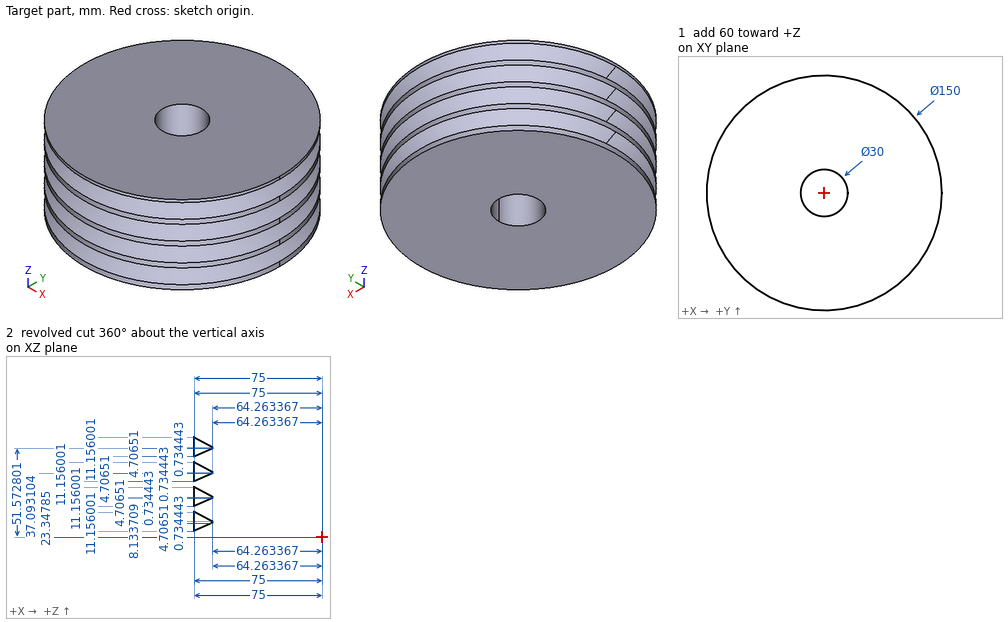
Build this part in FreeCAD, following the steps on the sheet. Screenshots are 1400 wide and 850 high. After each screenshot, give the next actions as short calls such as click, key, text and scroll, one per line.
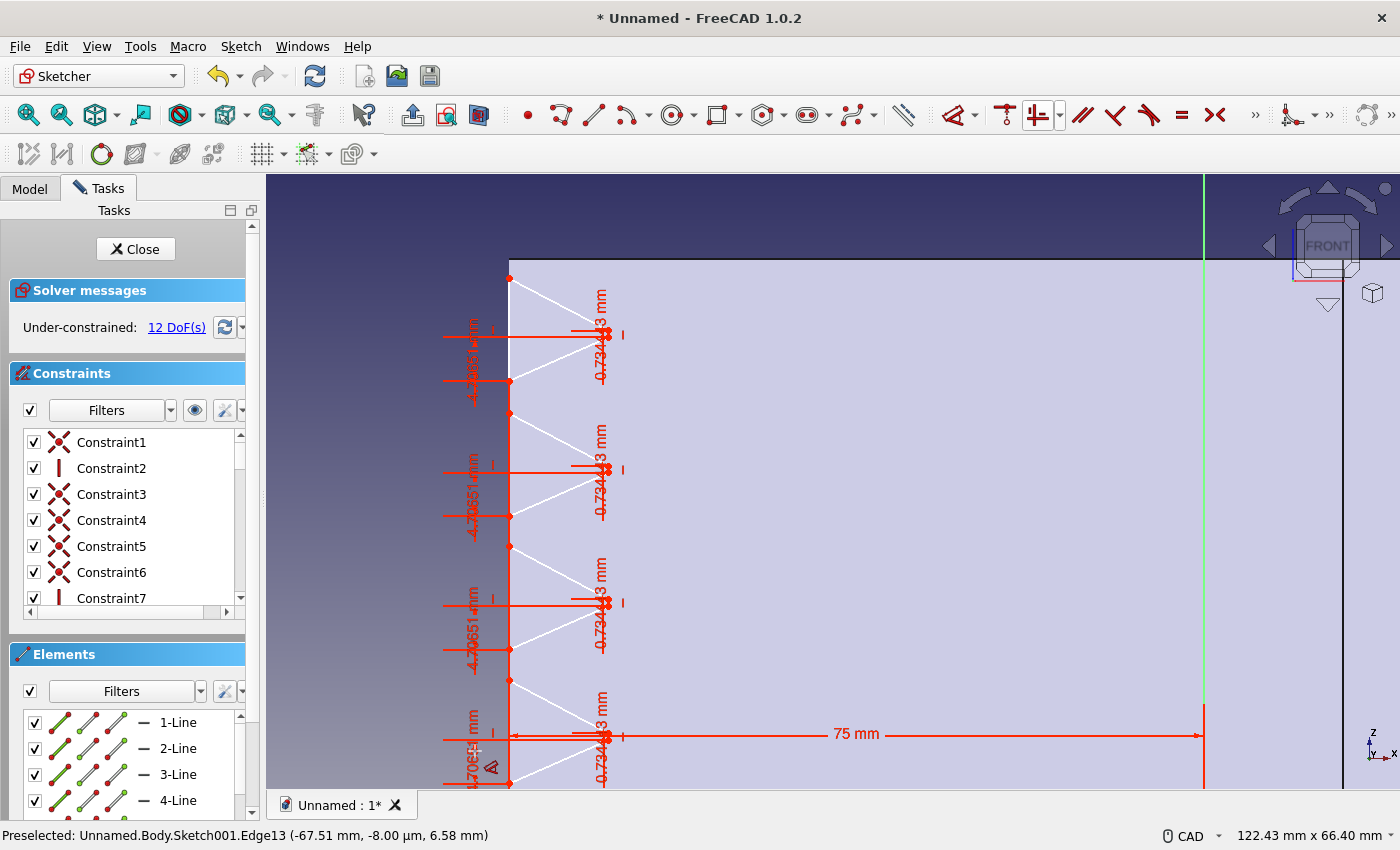
click(509, 350)
click(475, 330)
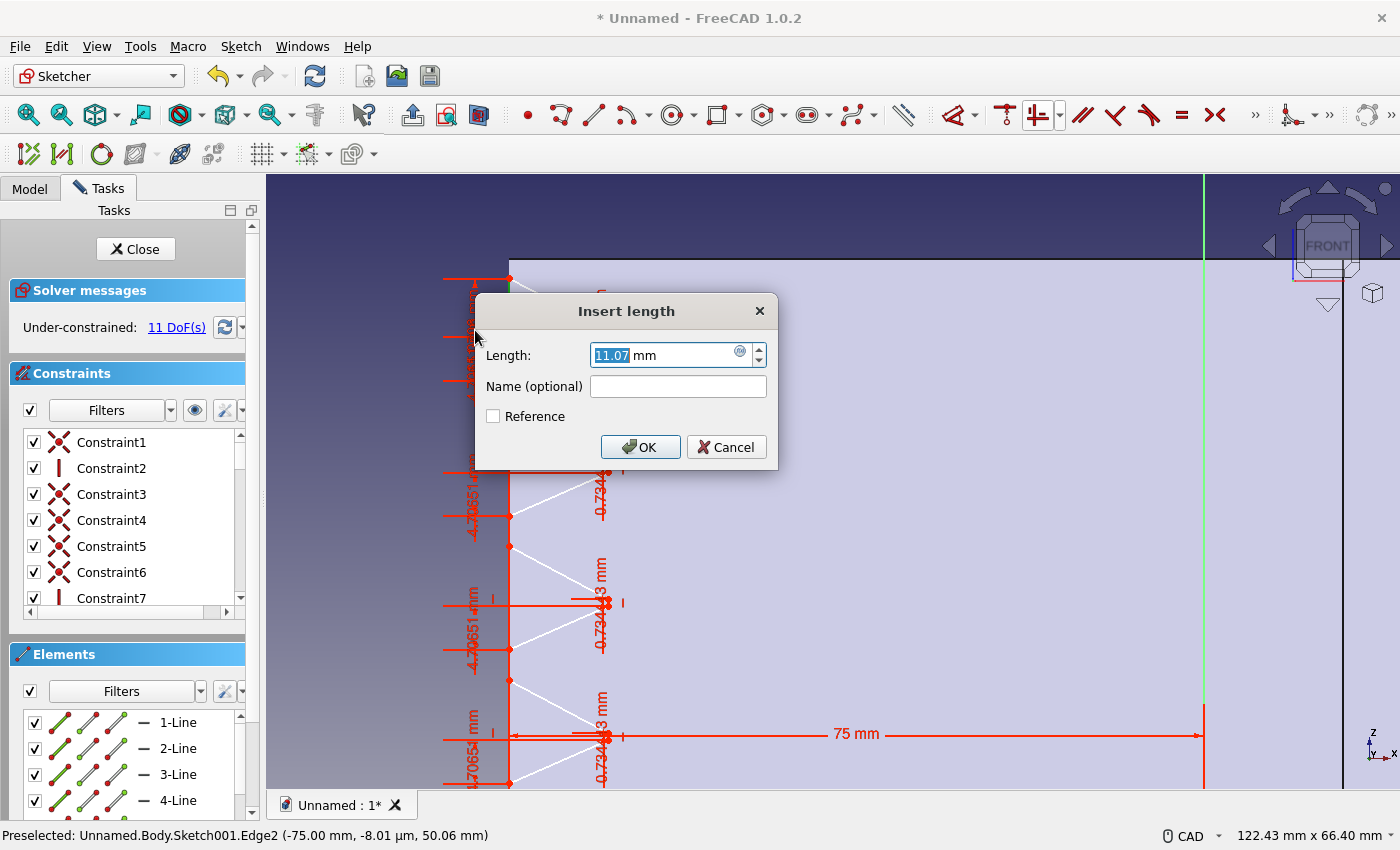
text(11.156001)
key(Return)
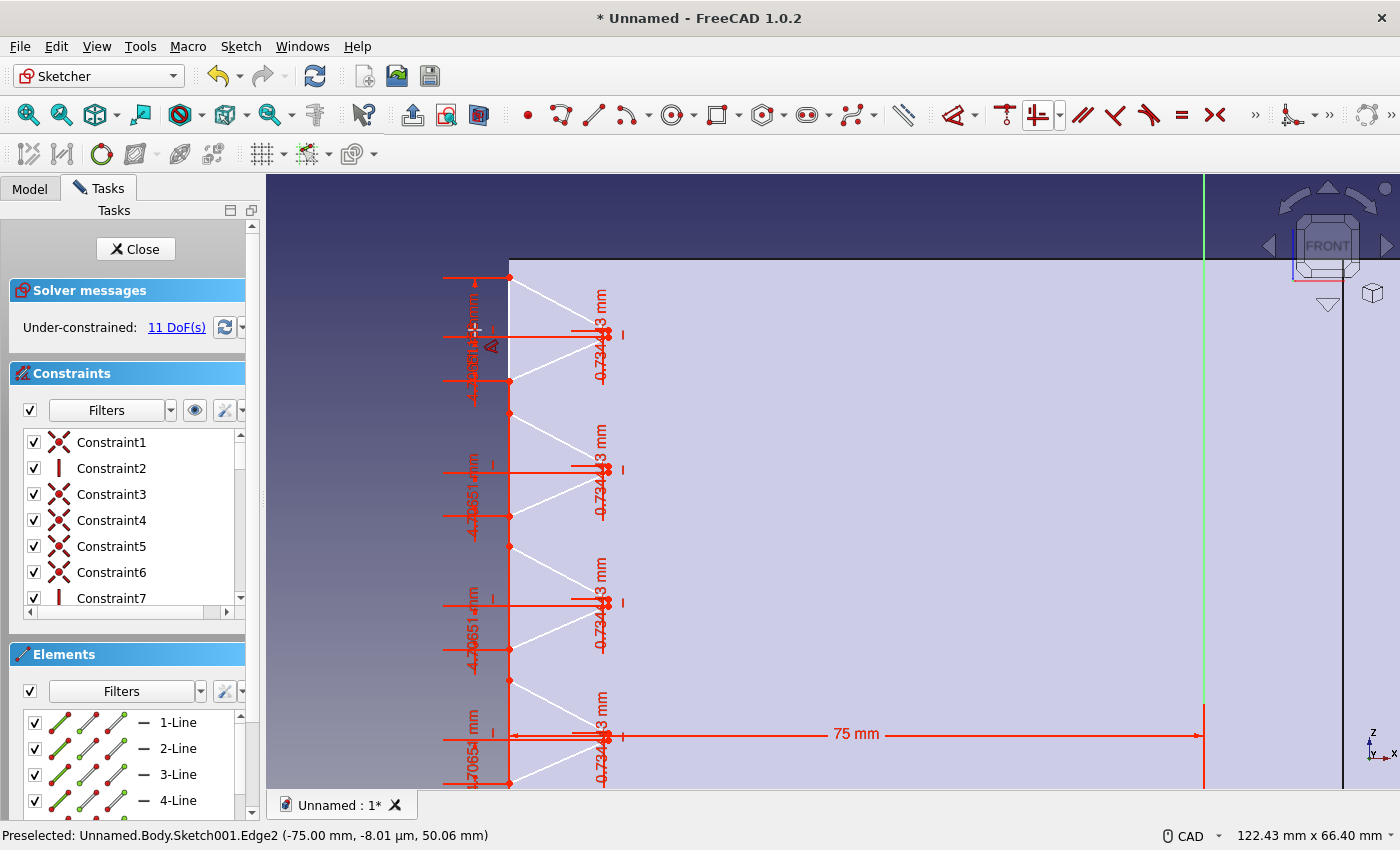
click(509, 486)
click(475, 465)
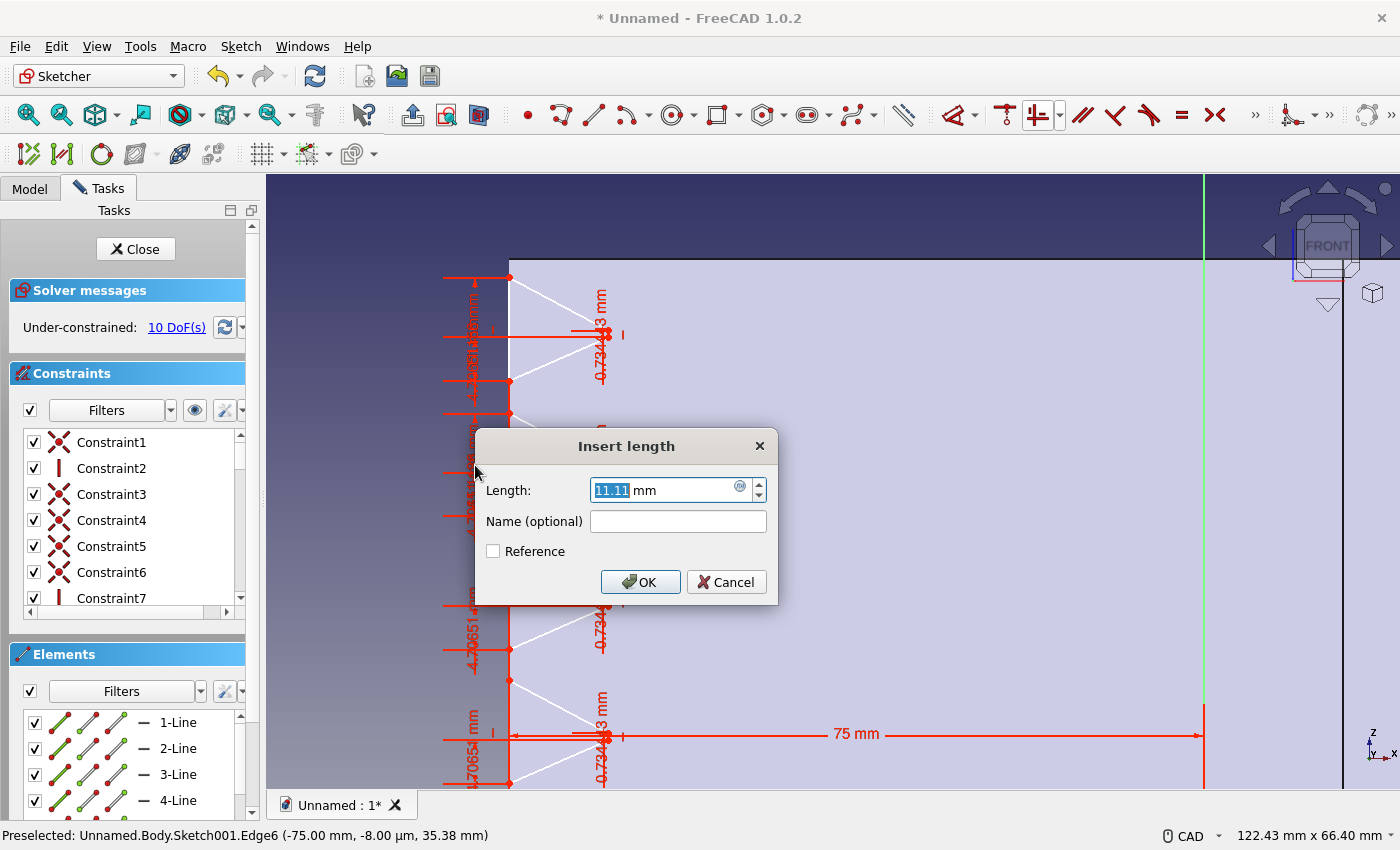
text(11.156001)
key(Return)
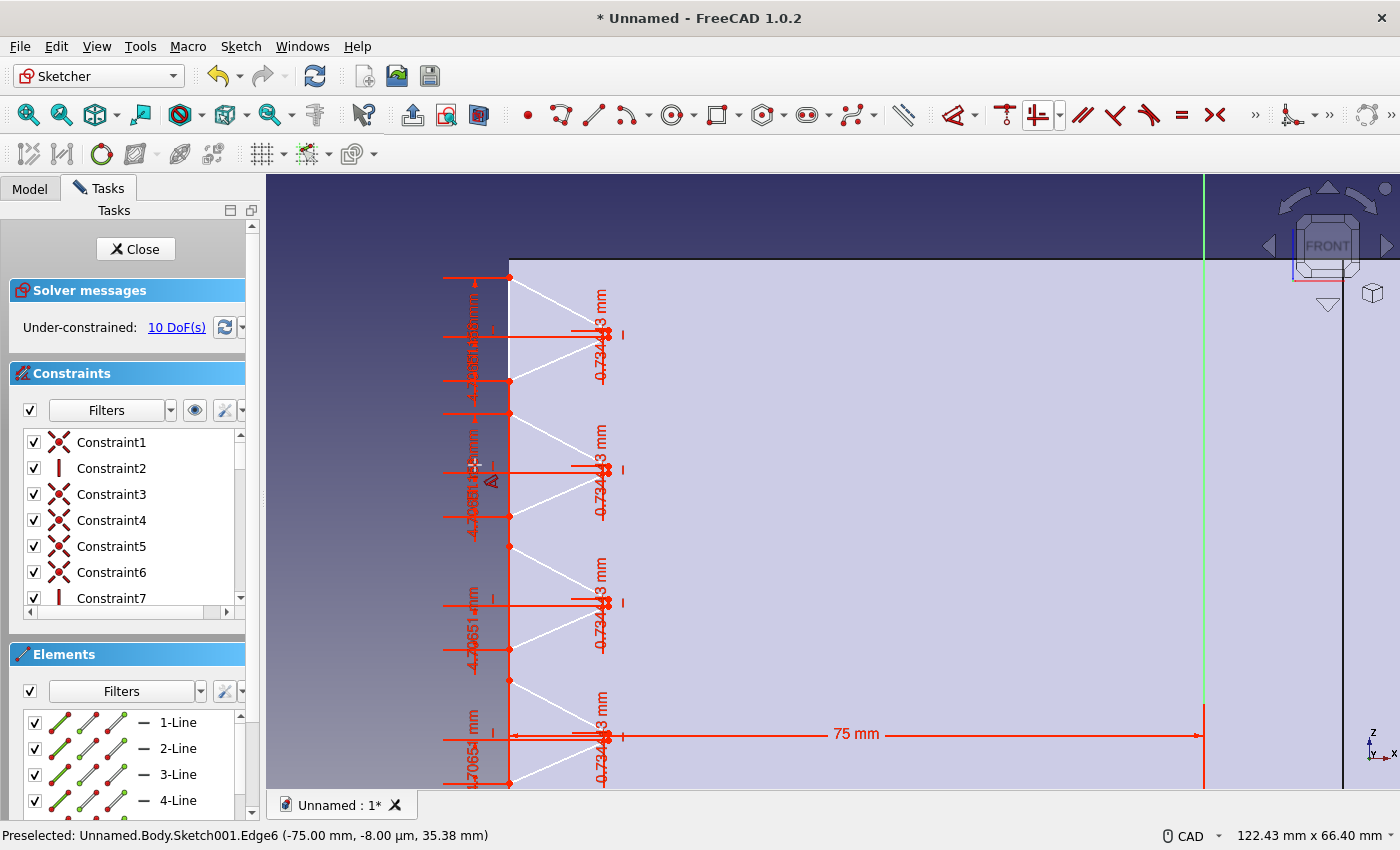
click(509, 619)
click(475, 598)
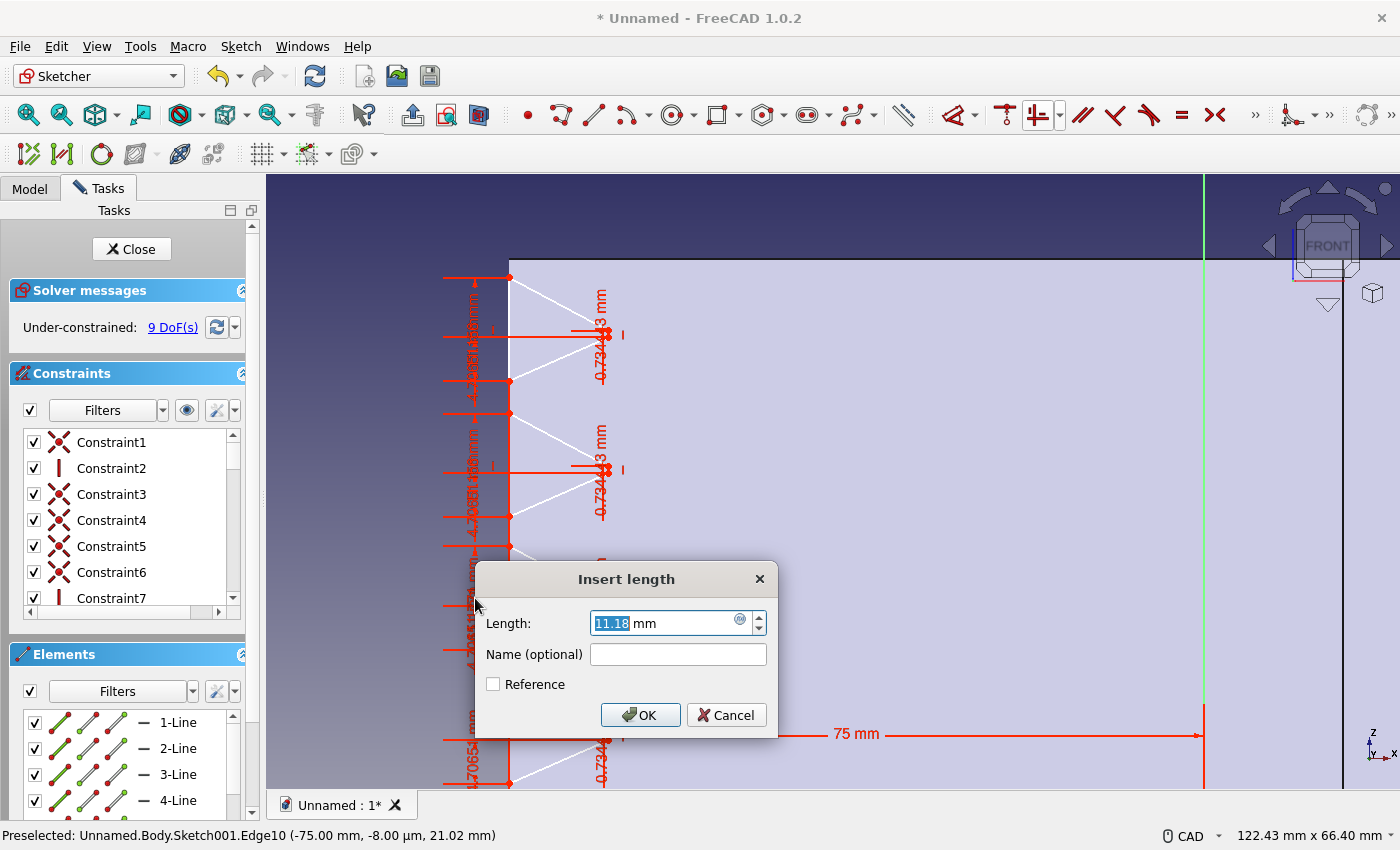
text(11.156001)
key(Return)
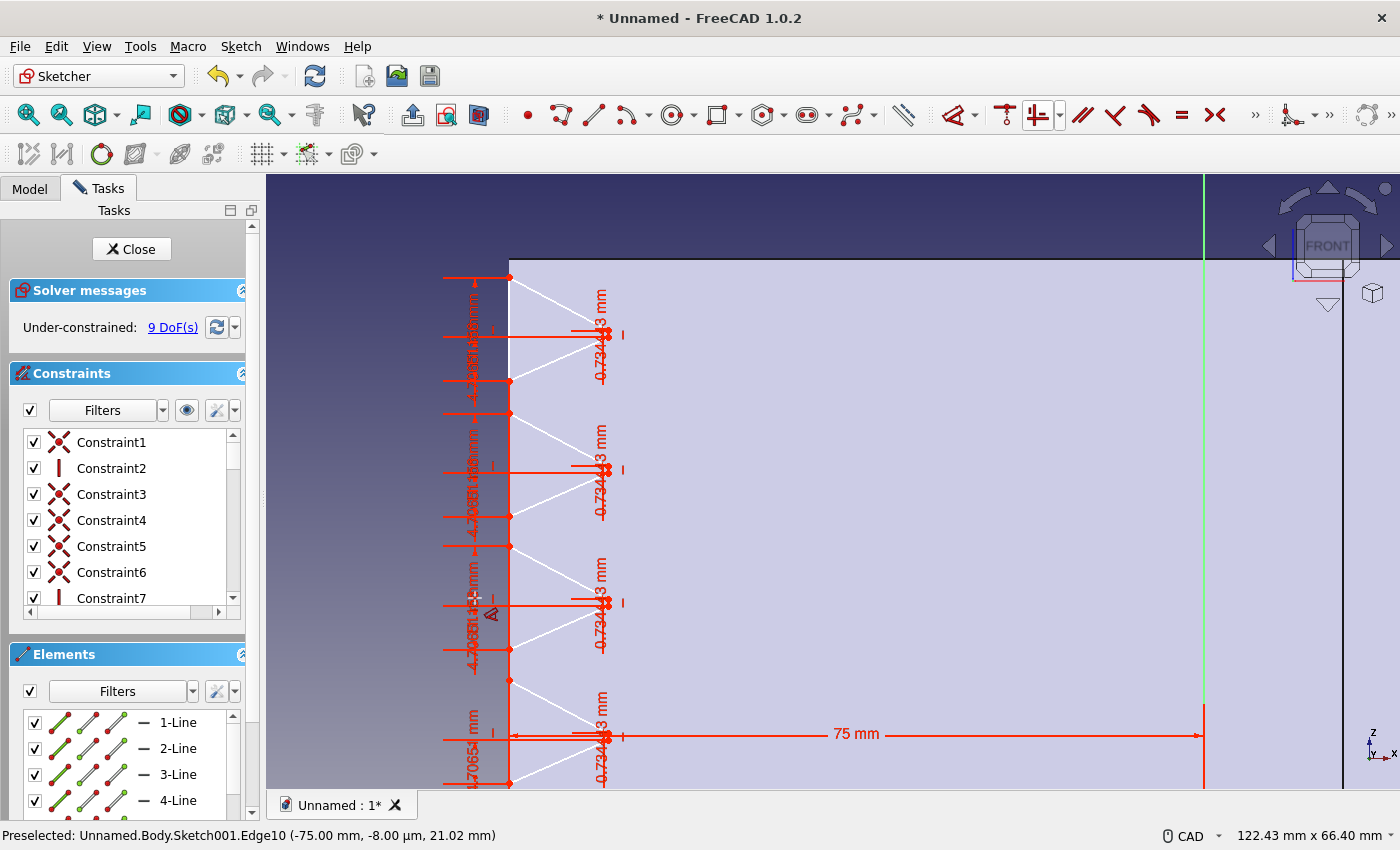
click(509, 753)
click(475, 721)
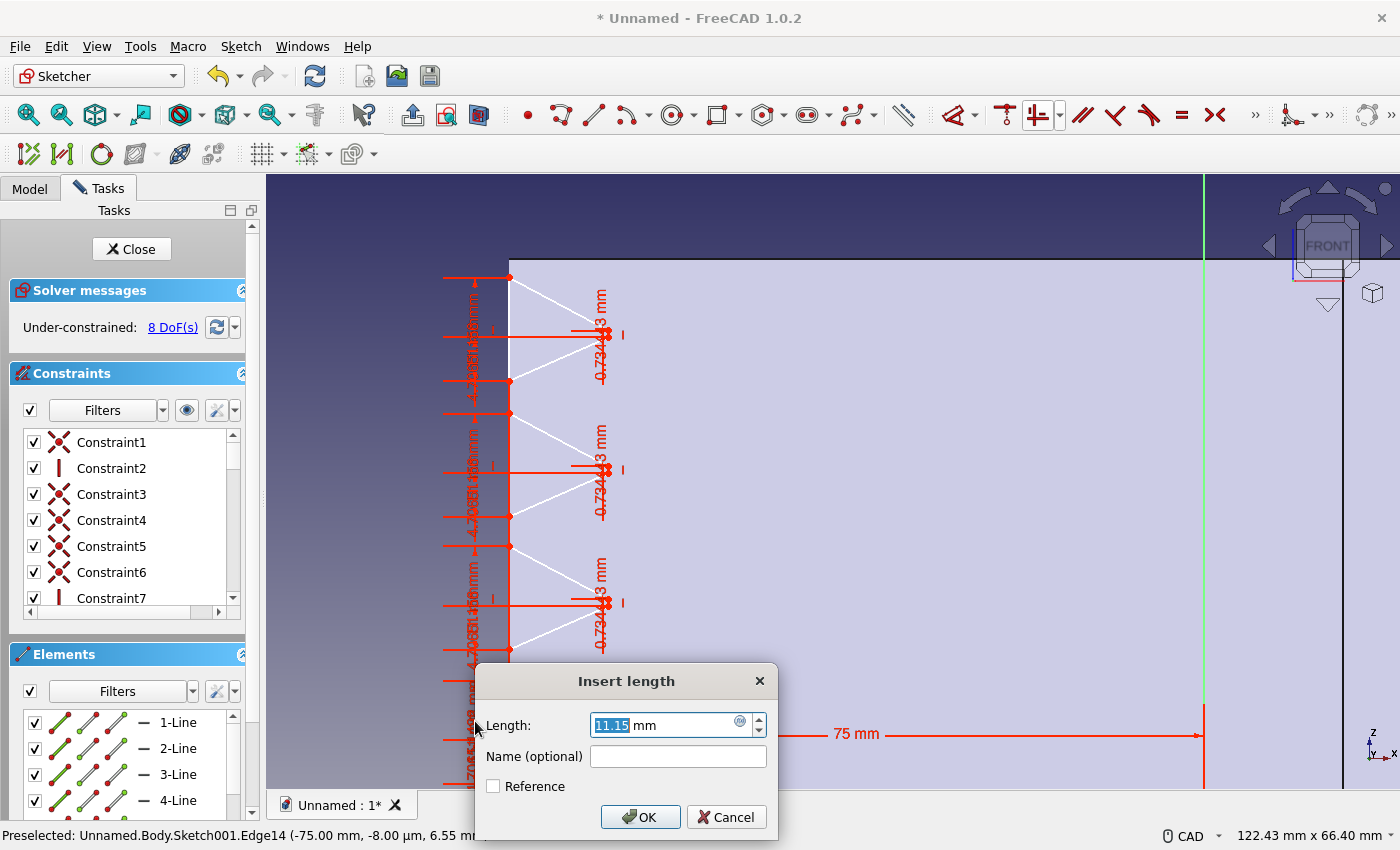
text(11.156001)
key(Return)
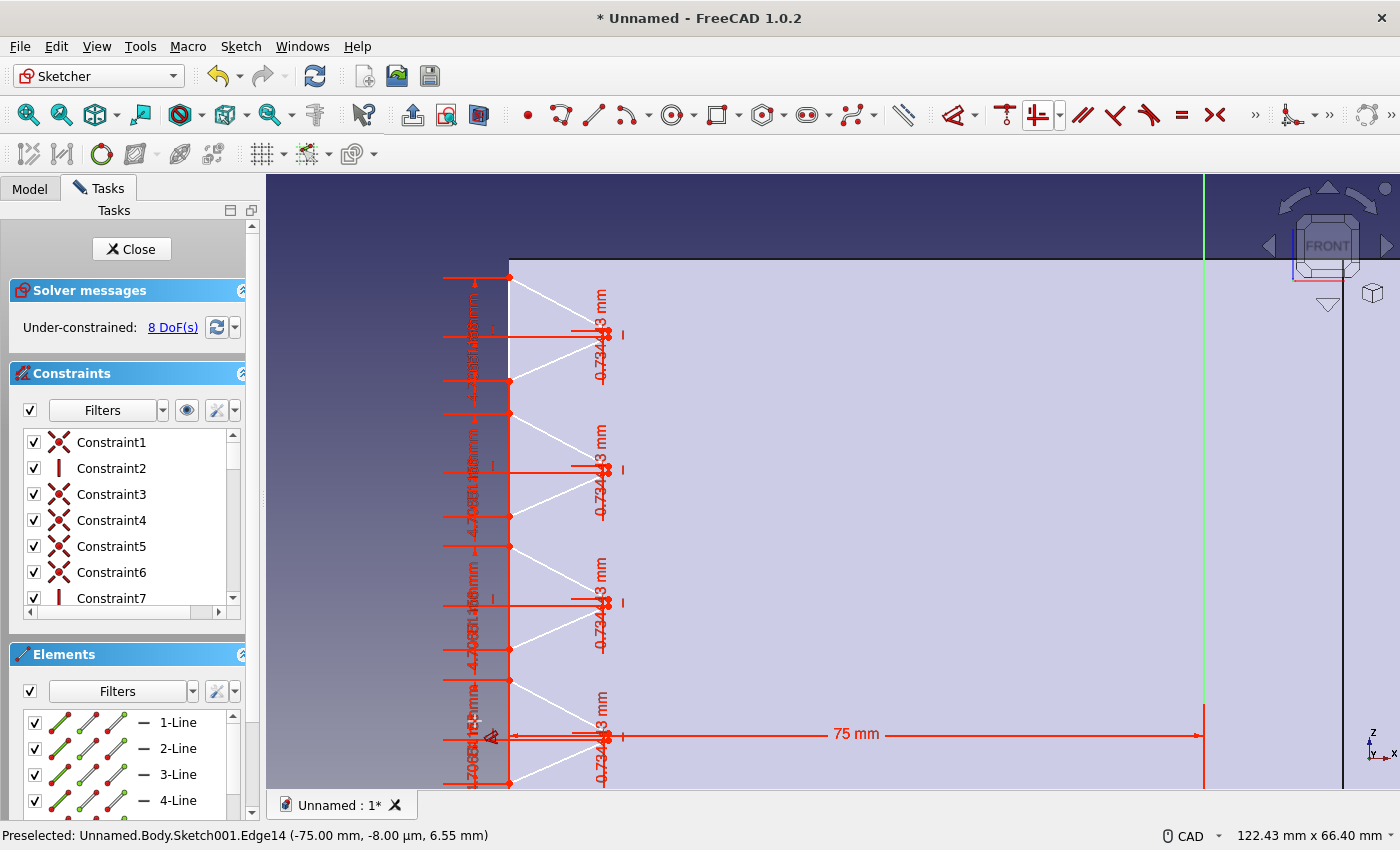
scroll(608, 599, up, 3)